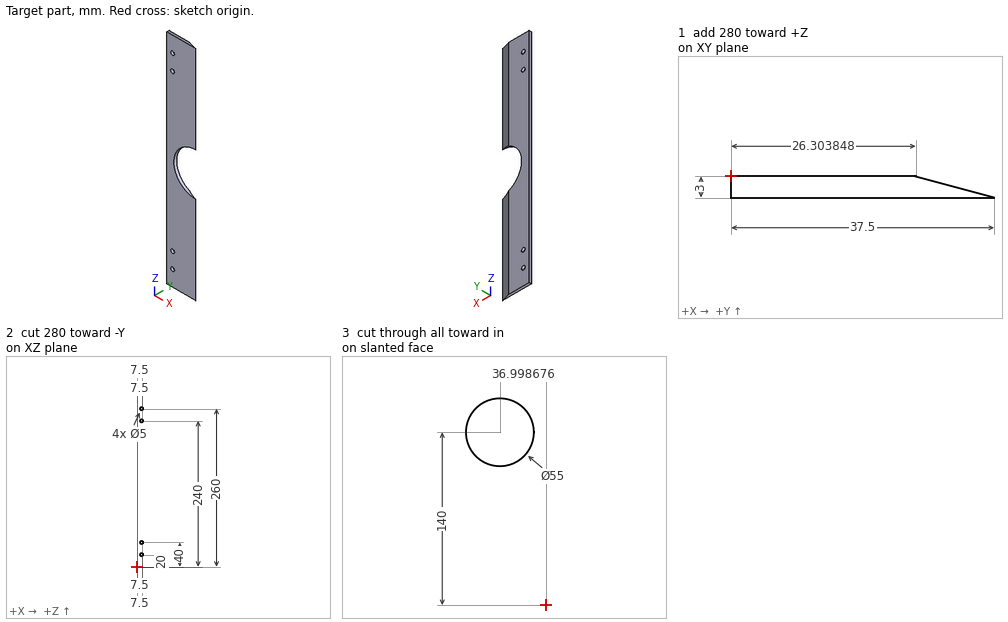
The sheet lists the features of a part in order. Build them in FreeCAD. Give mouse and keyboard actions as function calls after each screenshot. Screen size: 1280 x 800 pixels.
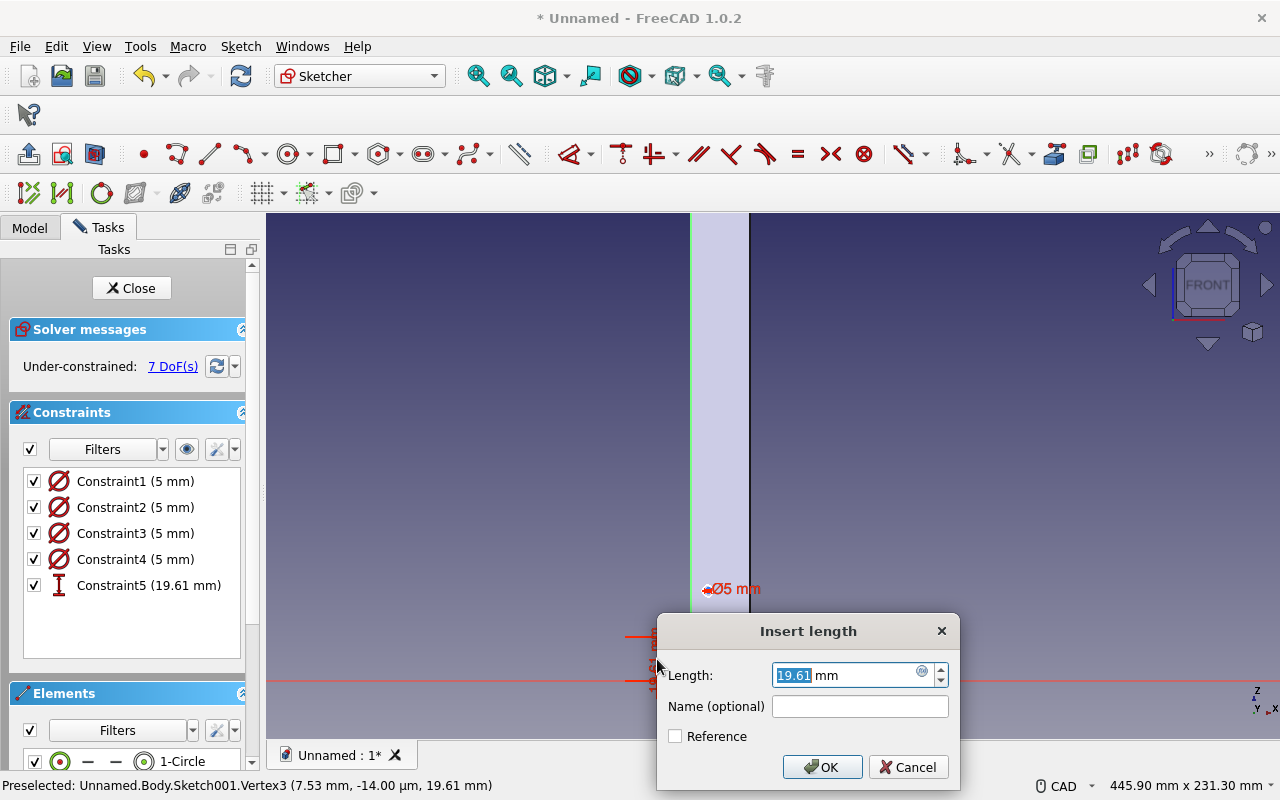
text(20)
key(Return)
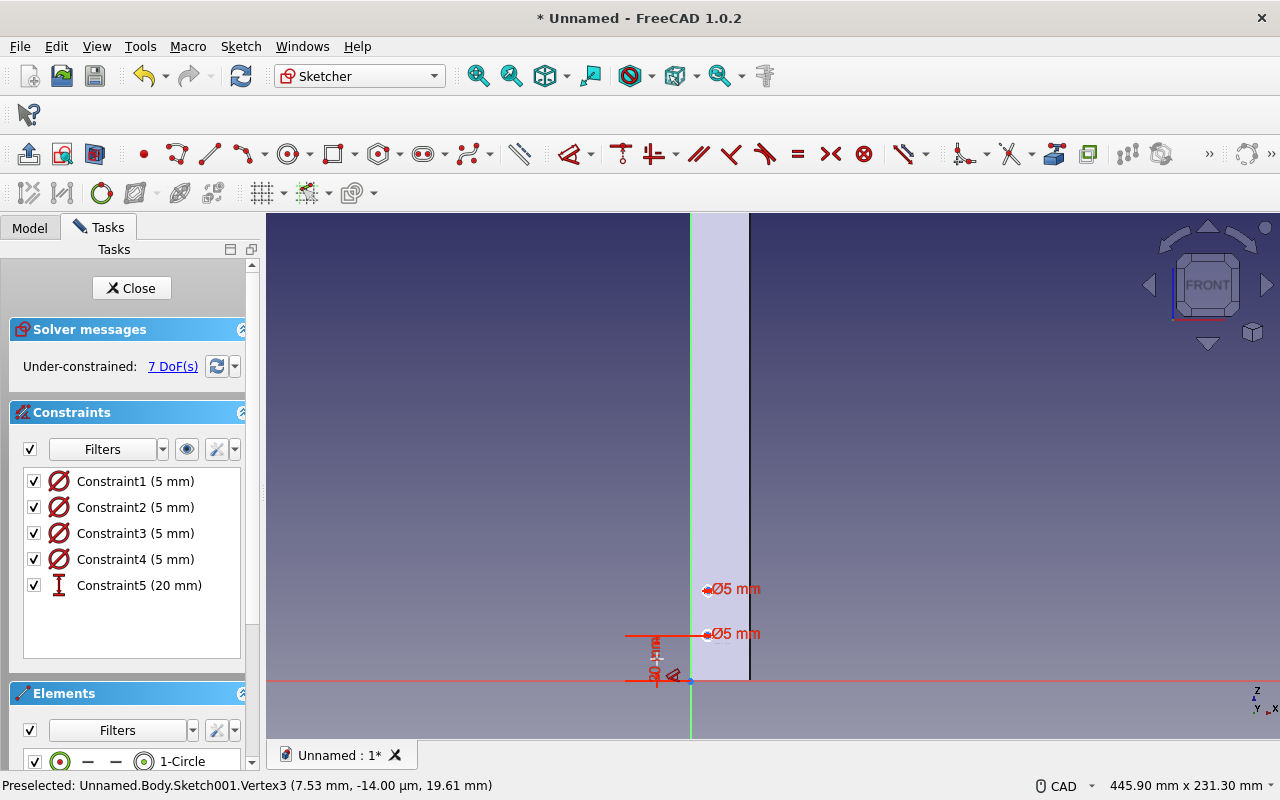
click(708, 591)
click(657, 636)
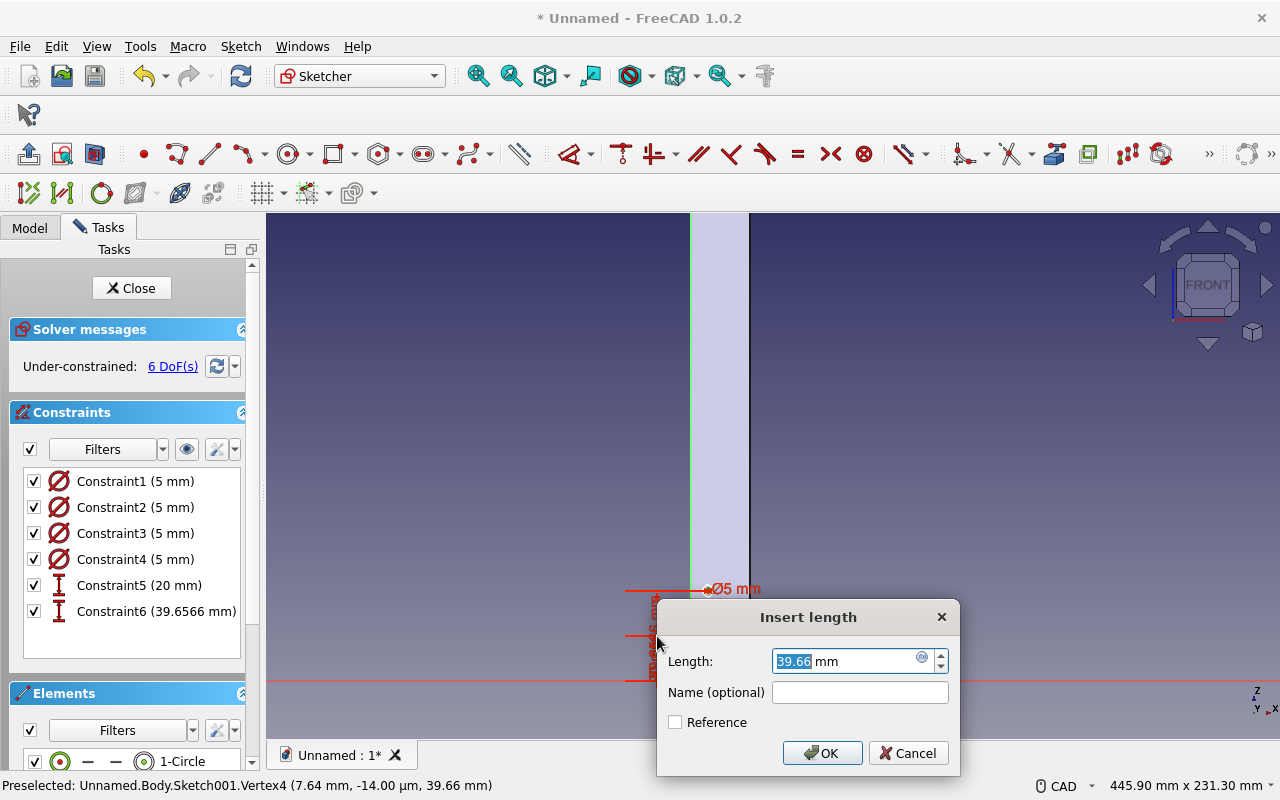
text(40)
key(Return)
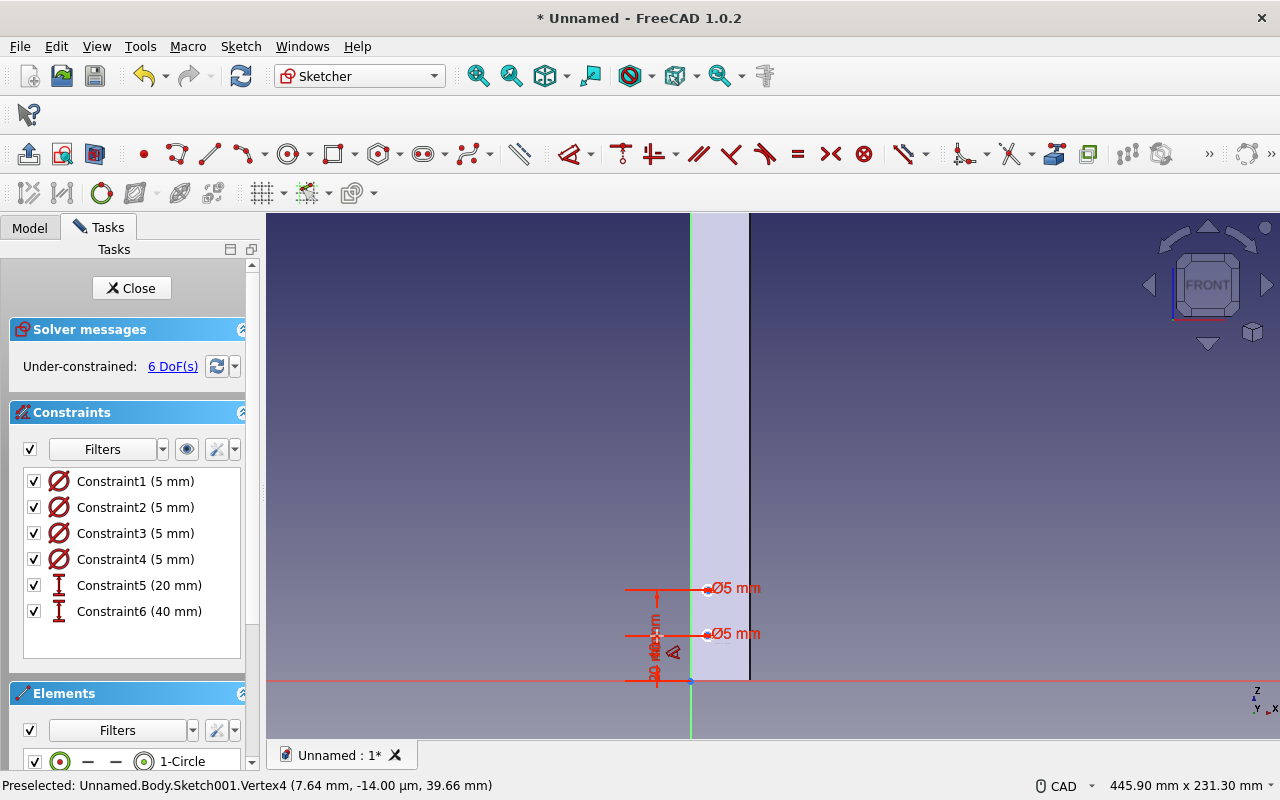
scroll(708, 589, down, 3)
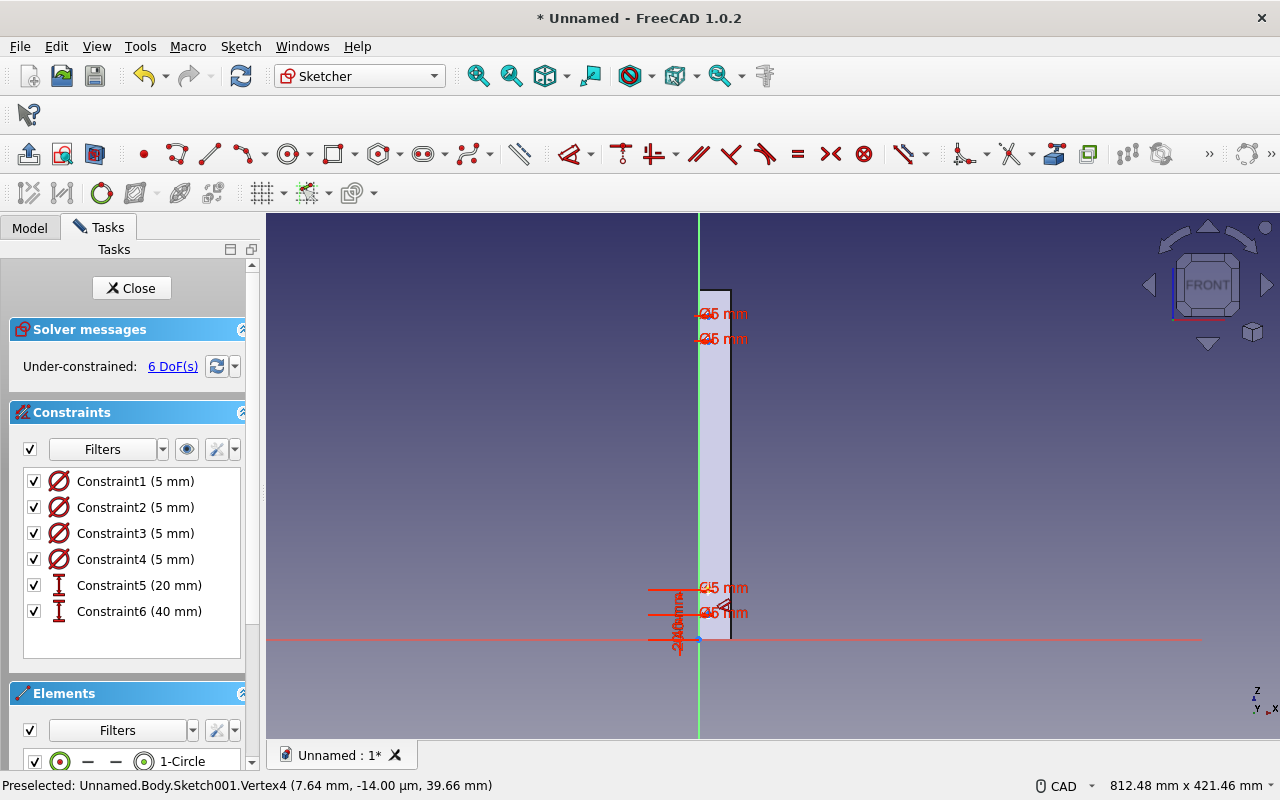
scroll(708, 316, up, 8)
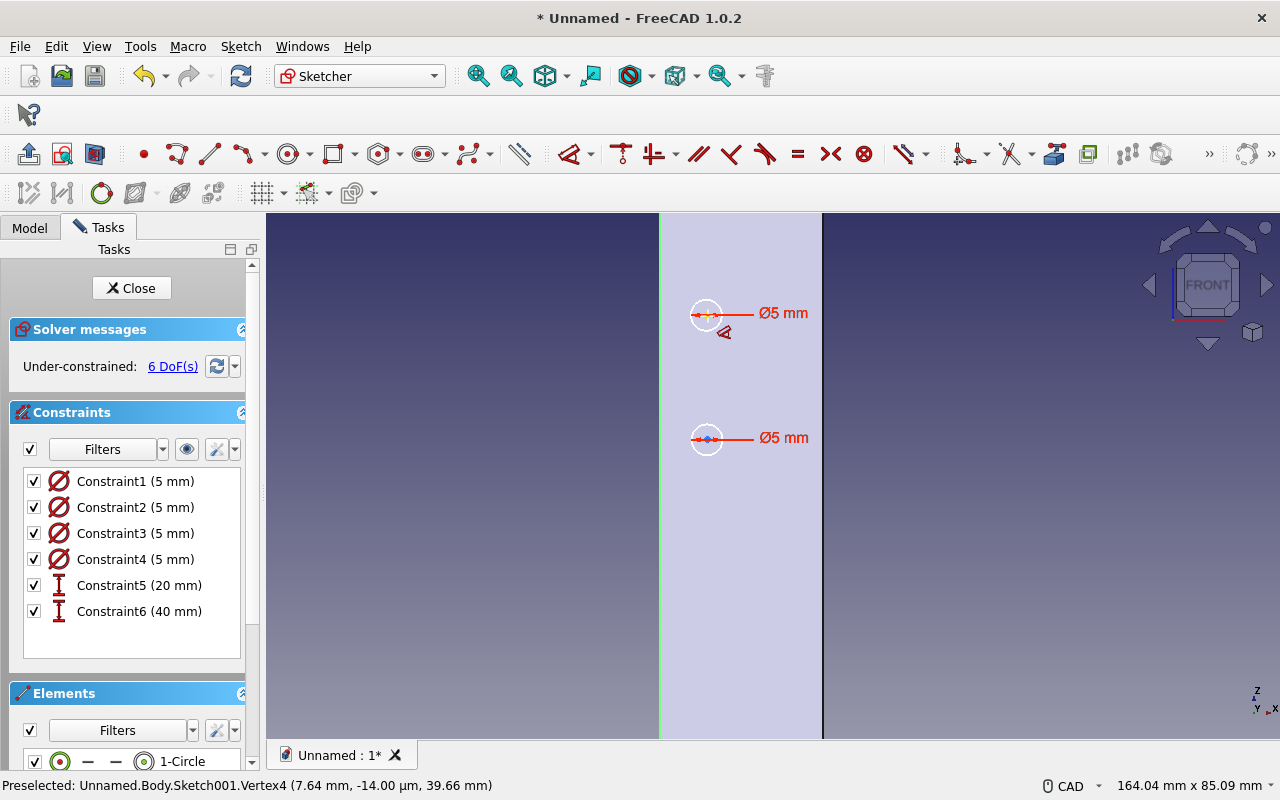
click(706, 315)
click(683, 281)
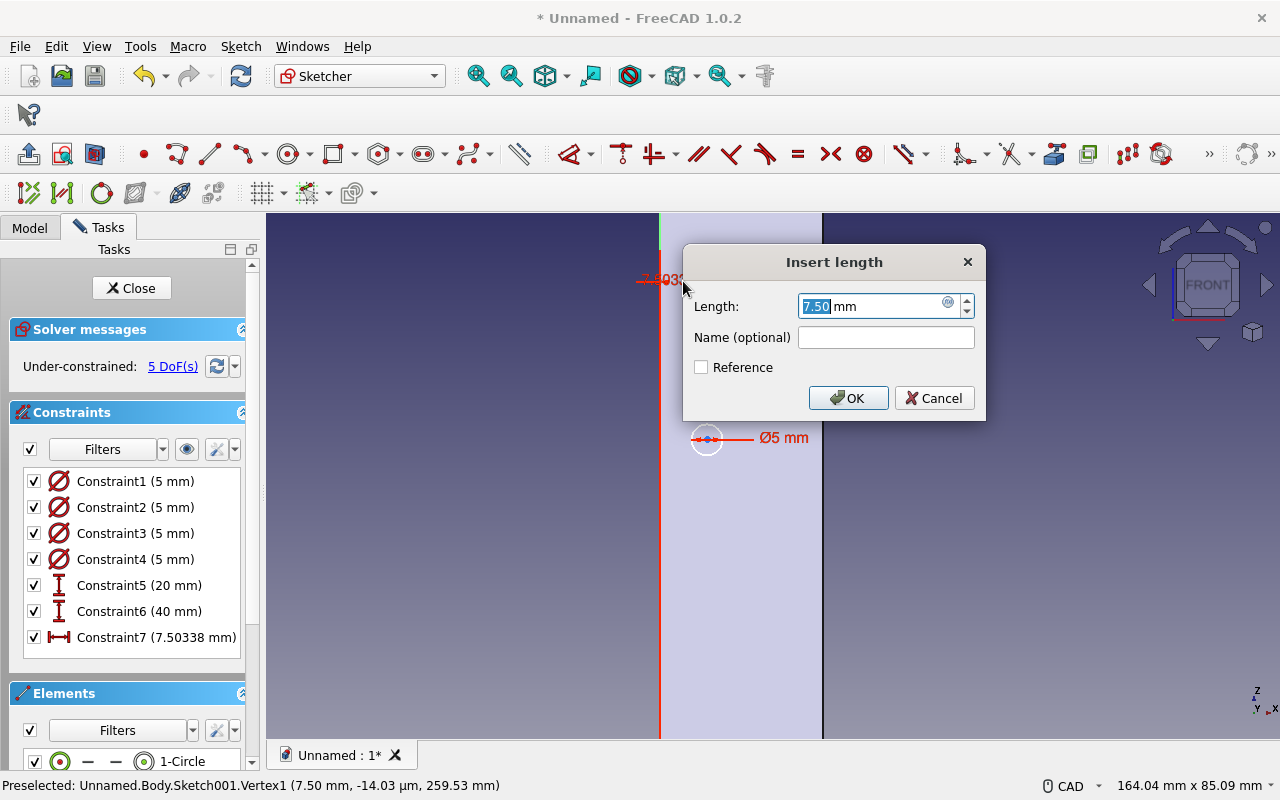
text(7.5)
key(Return)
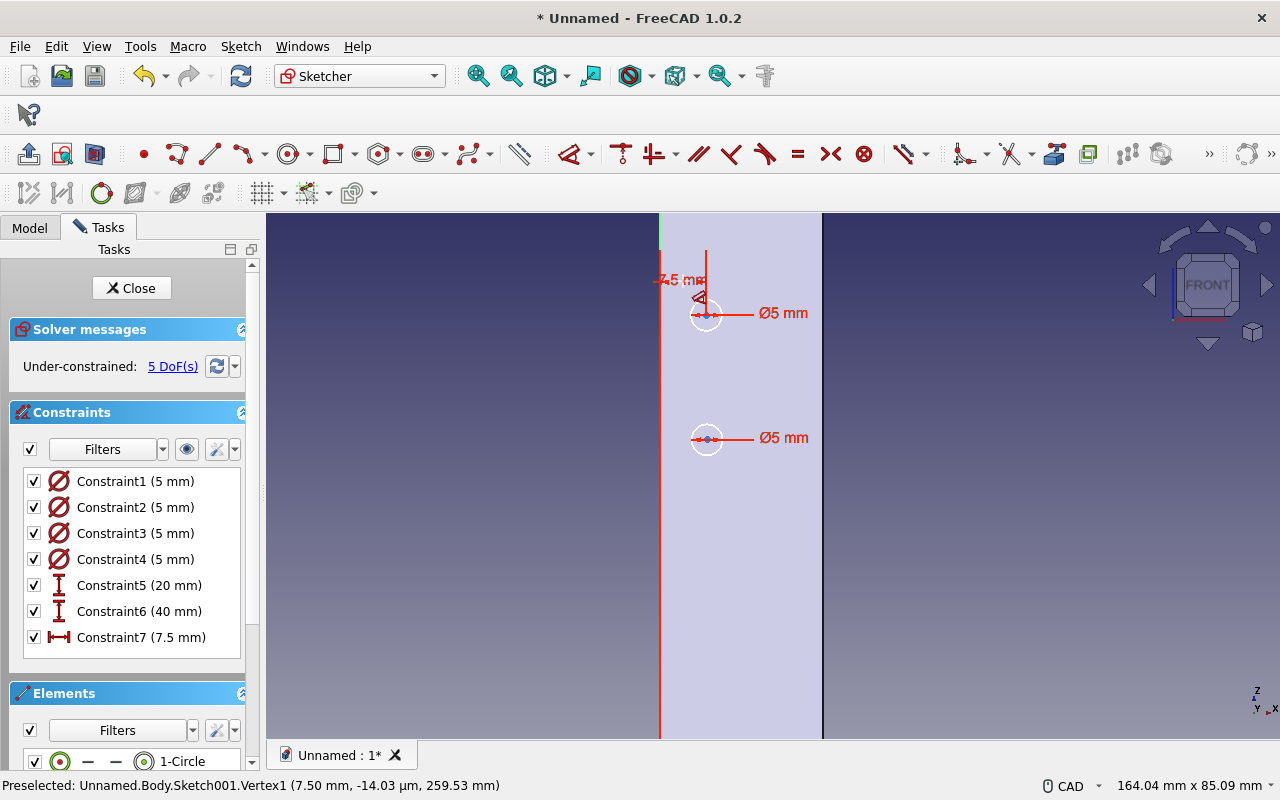
scroll(708, 316, down, 8)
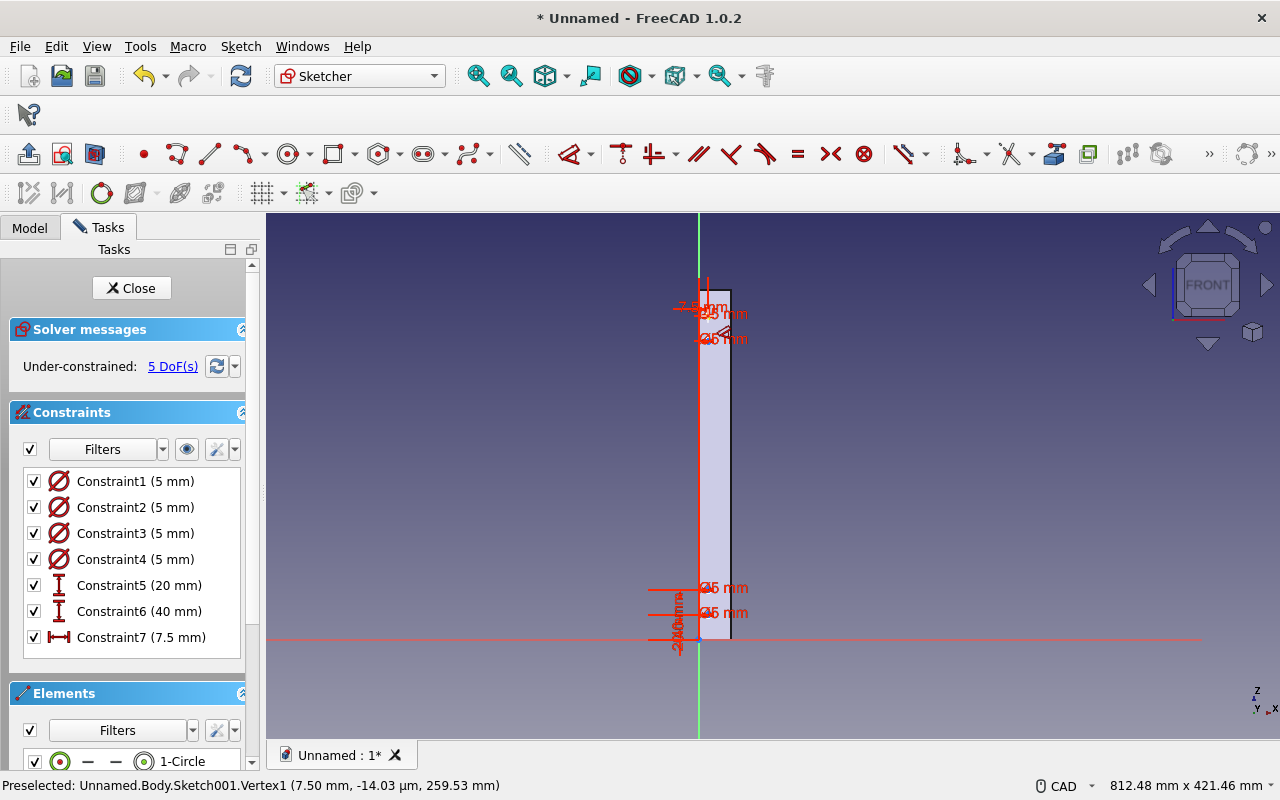
click(708, 316)
click(665, 478)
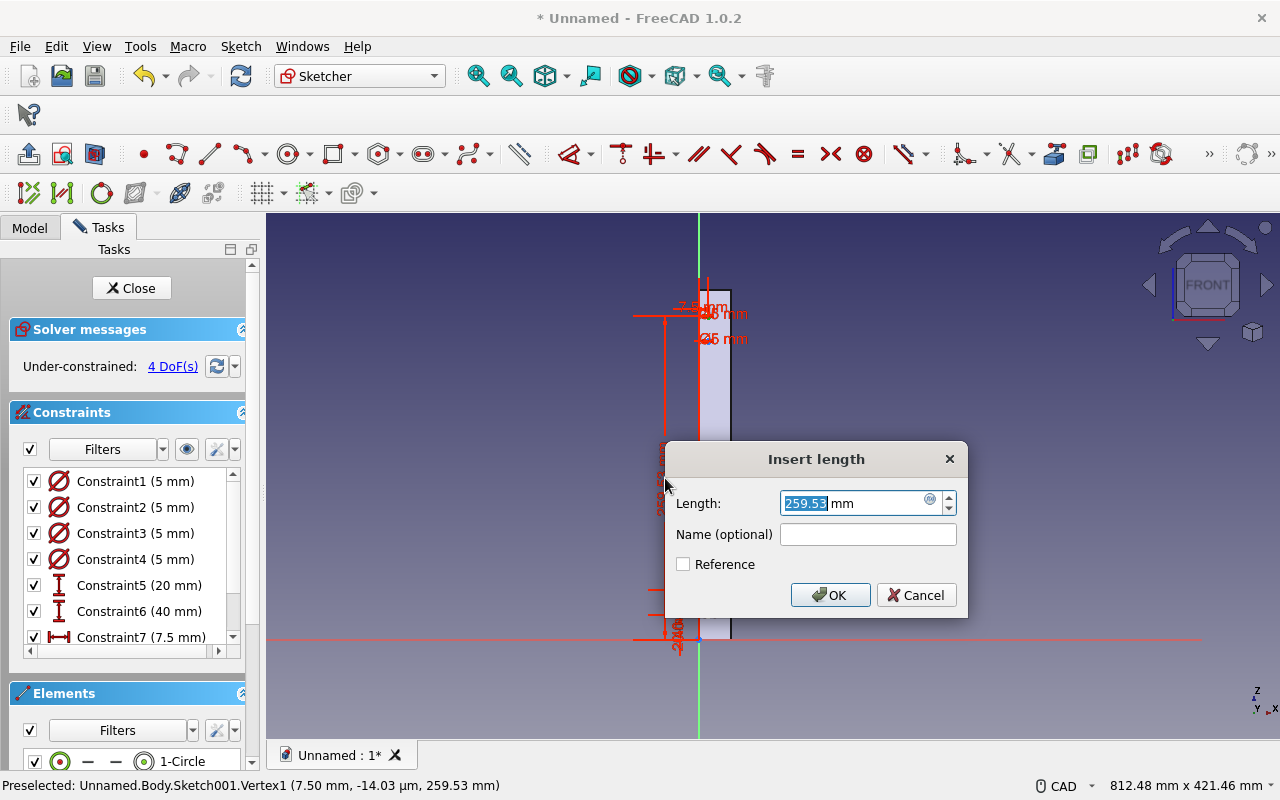
text(260)
key(Return)